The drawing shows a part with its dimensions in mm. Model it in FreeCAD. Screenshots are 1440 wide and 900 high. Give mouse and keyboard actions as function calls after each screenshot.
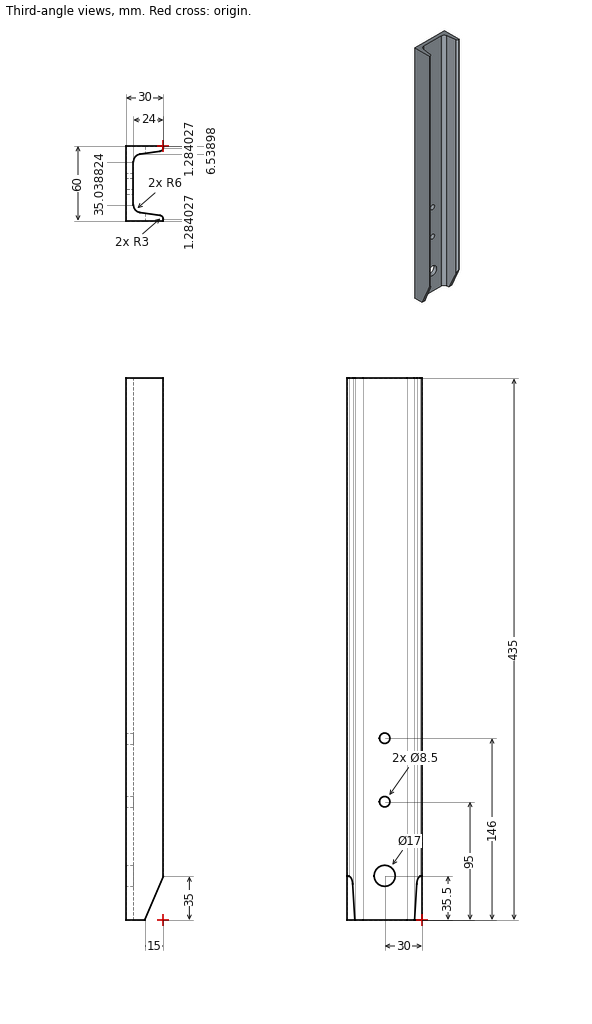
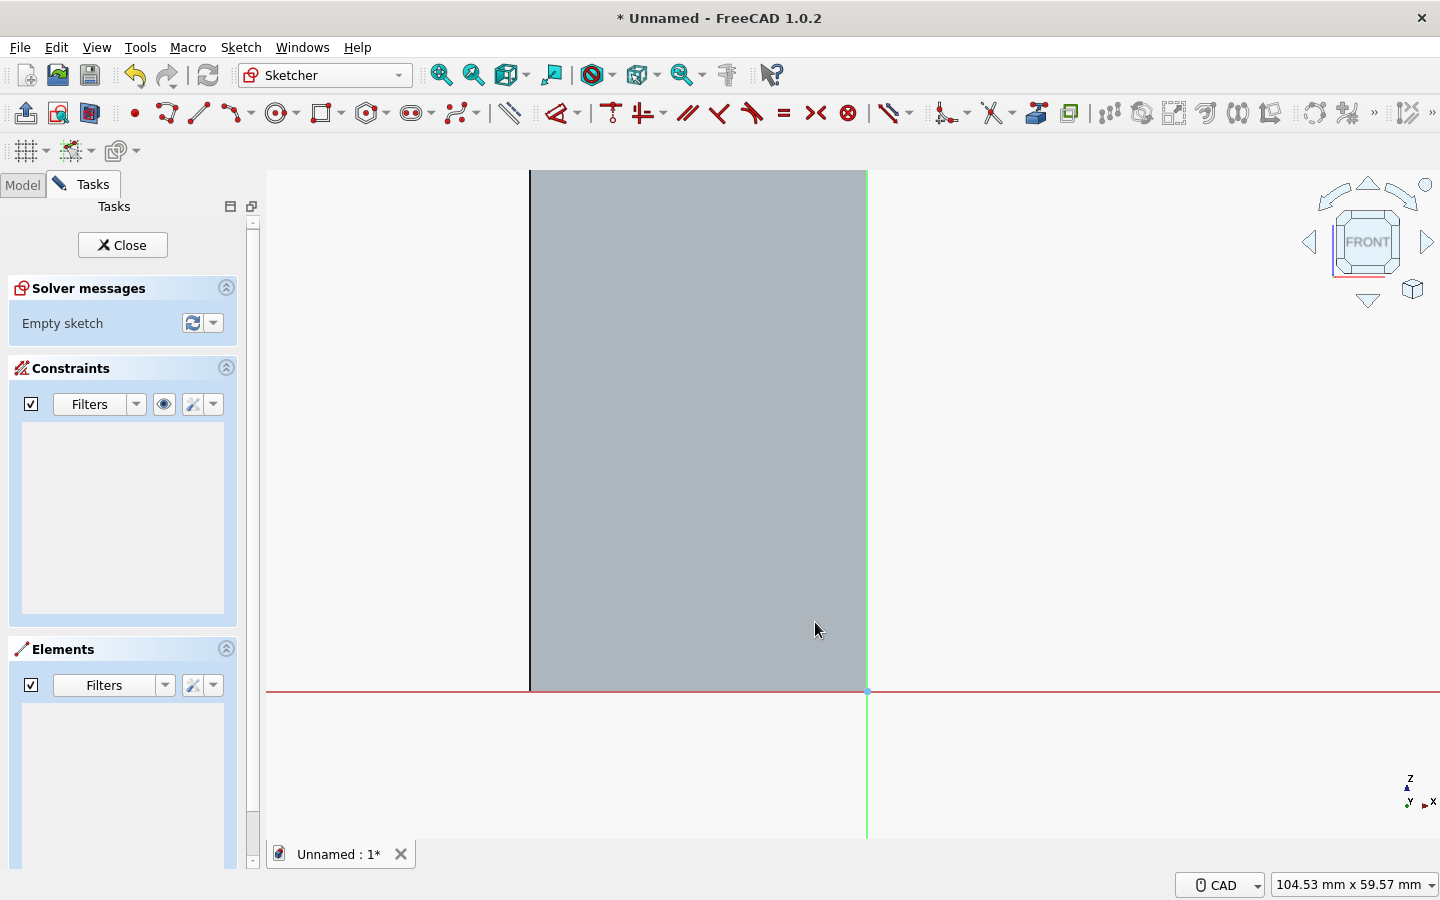
click(168, 114)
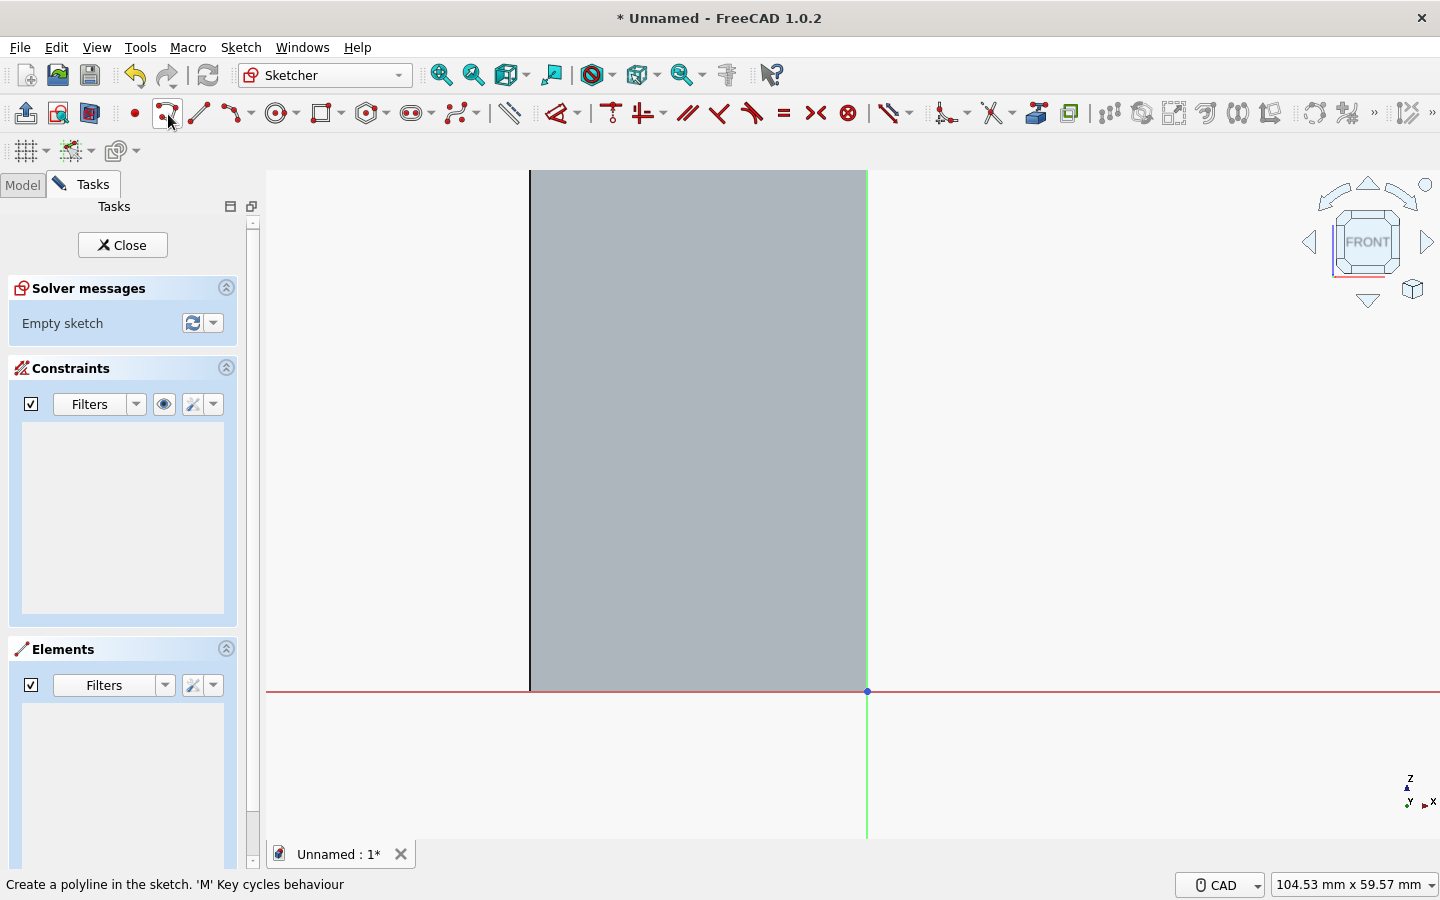
click(867, 692)
click(699, 683)
click(858, 299)
click(867, 692)
key(Escape)
key(Escape)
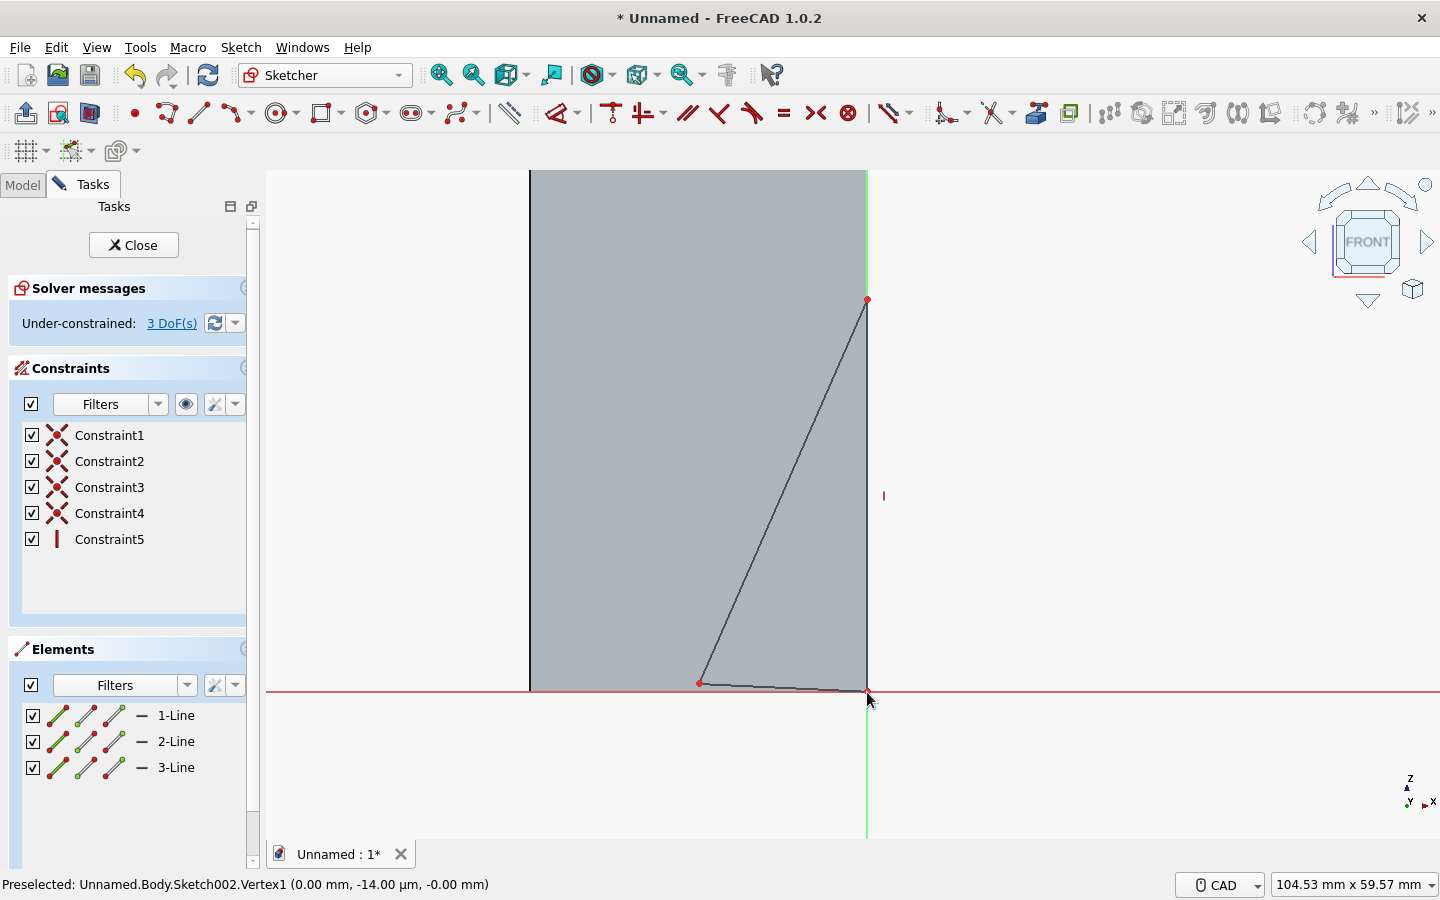
click(817, 689)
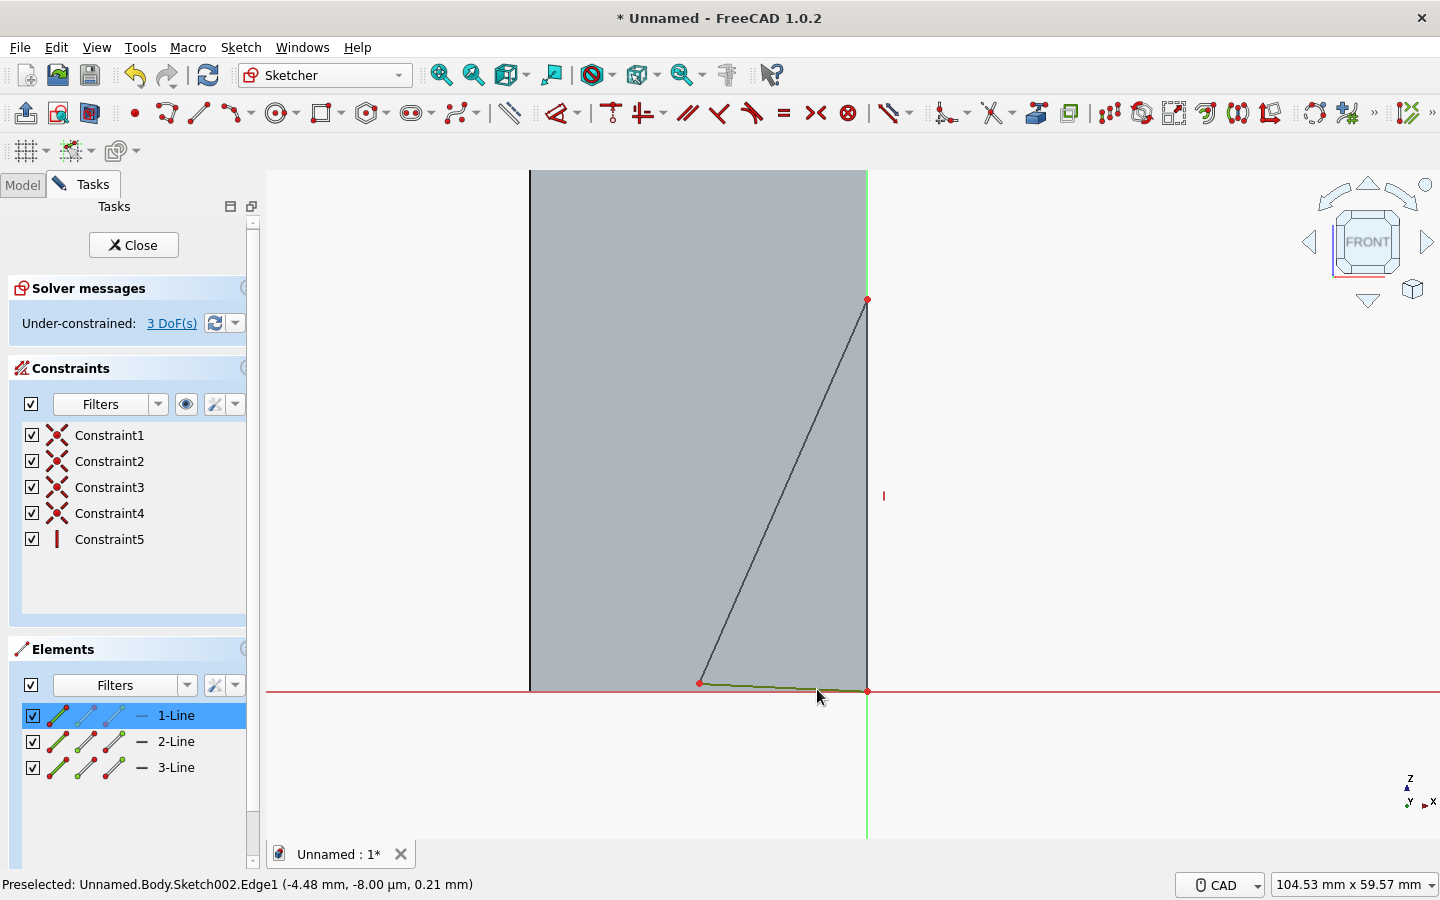
key(h)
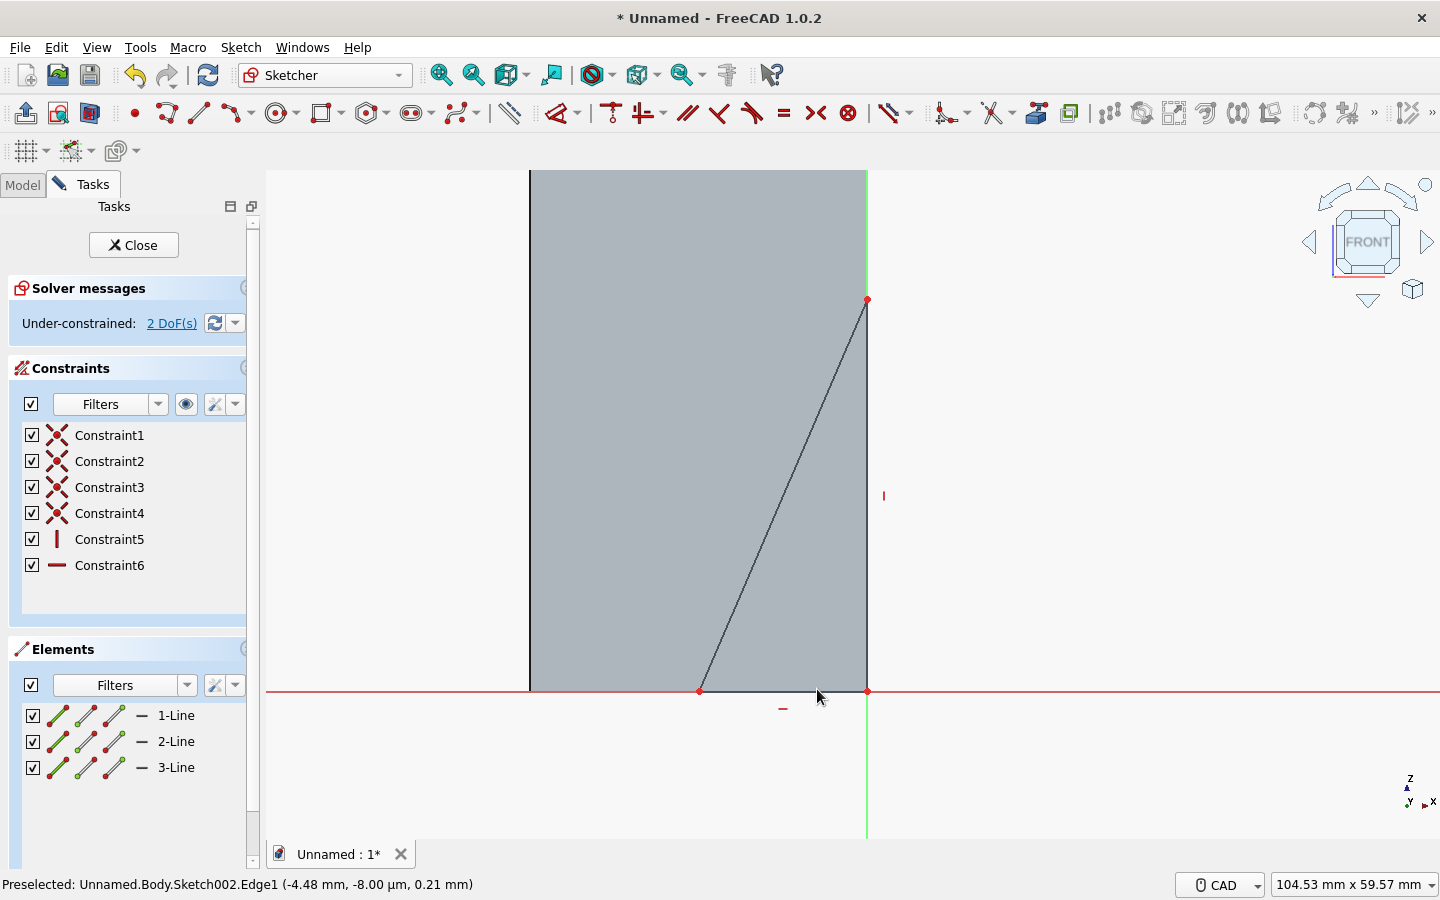
key(d)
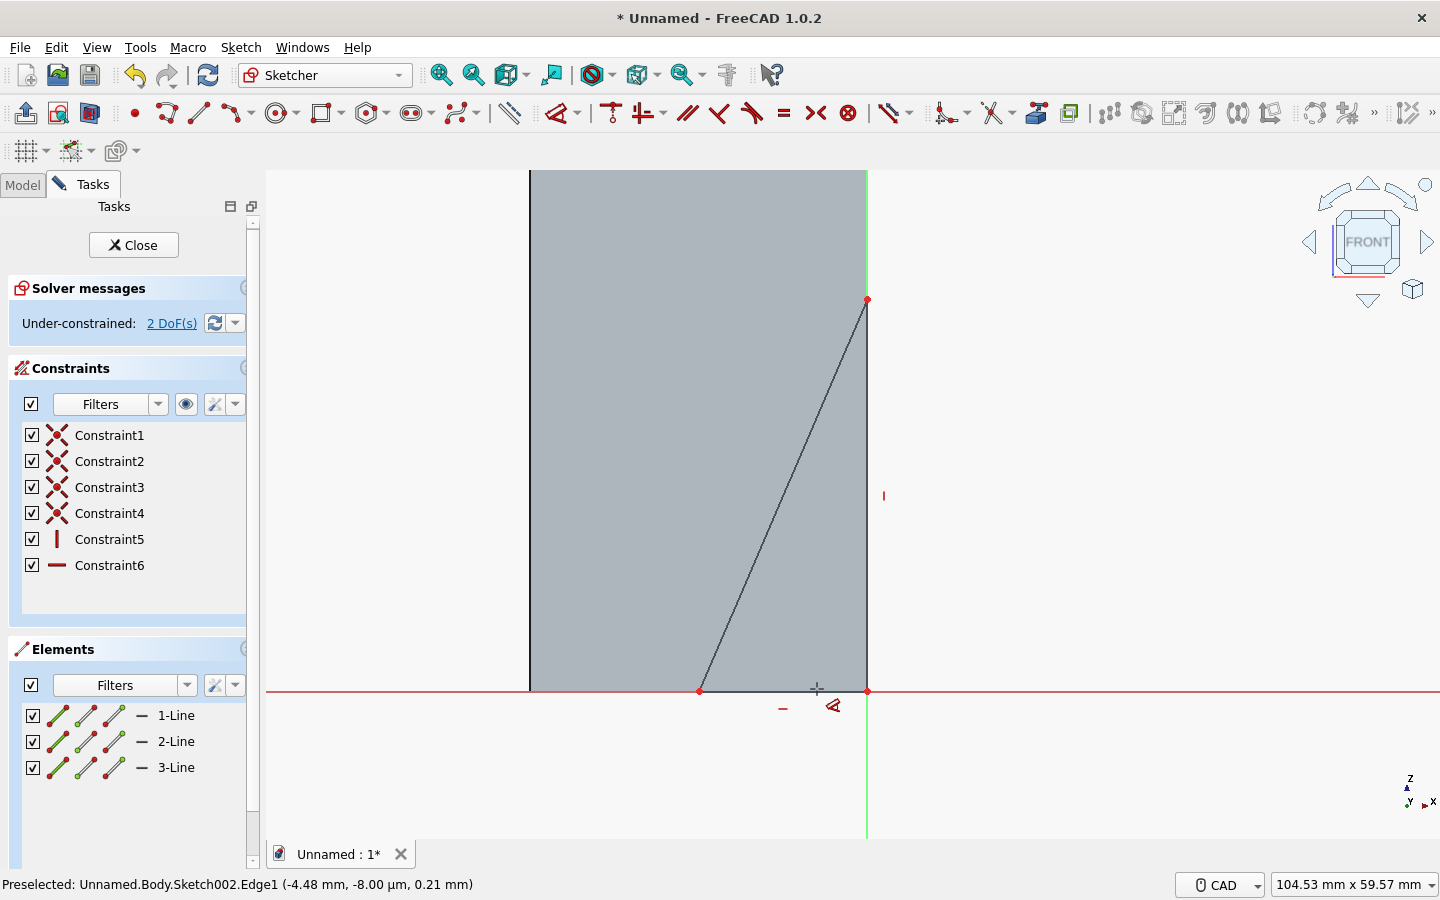
click(817, 692)
click(783, 726)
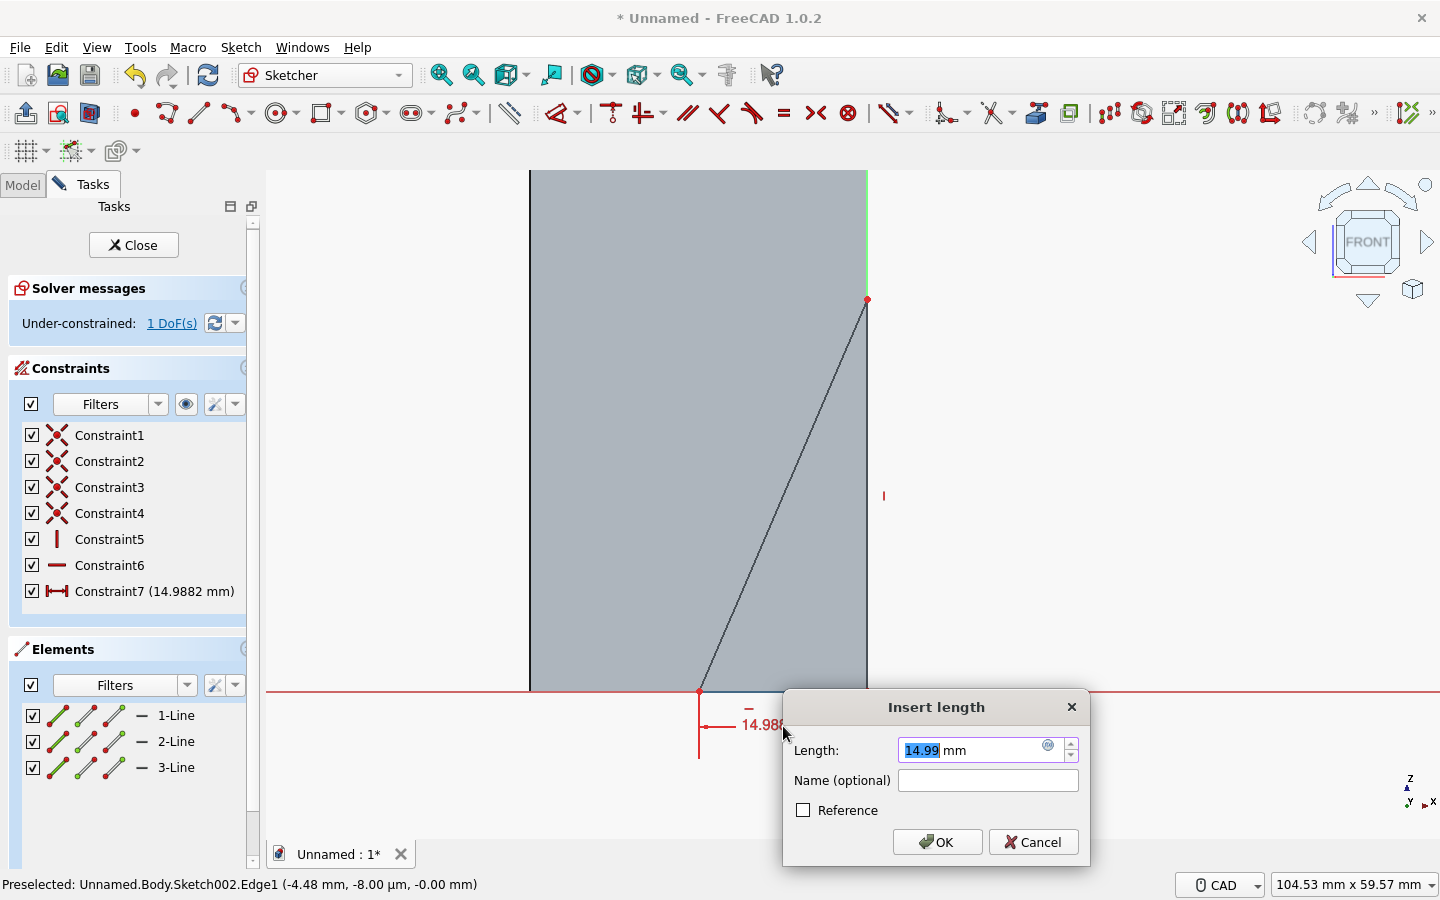
text(15)
key(Return)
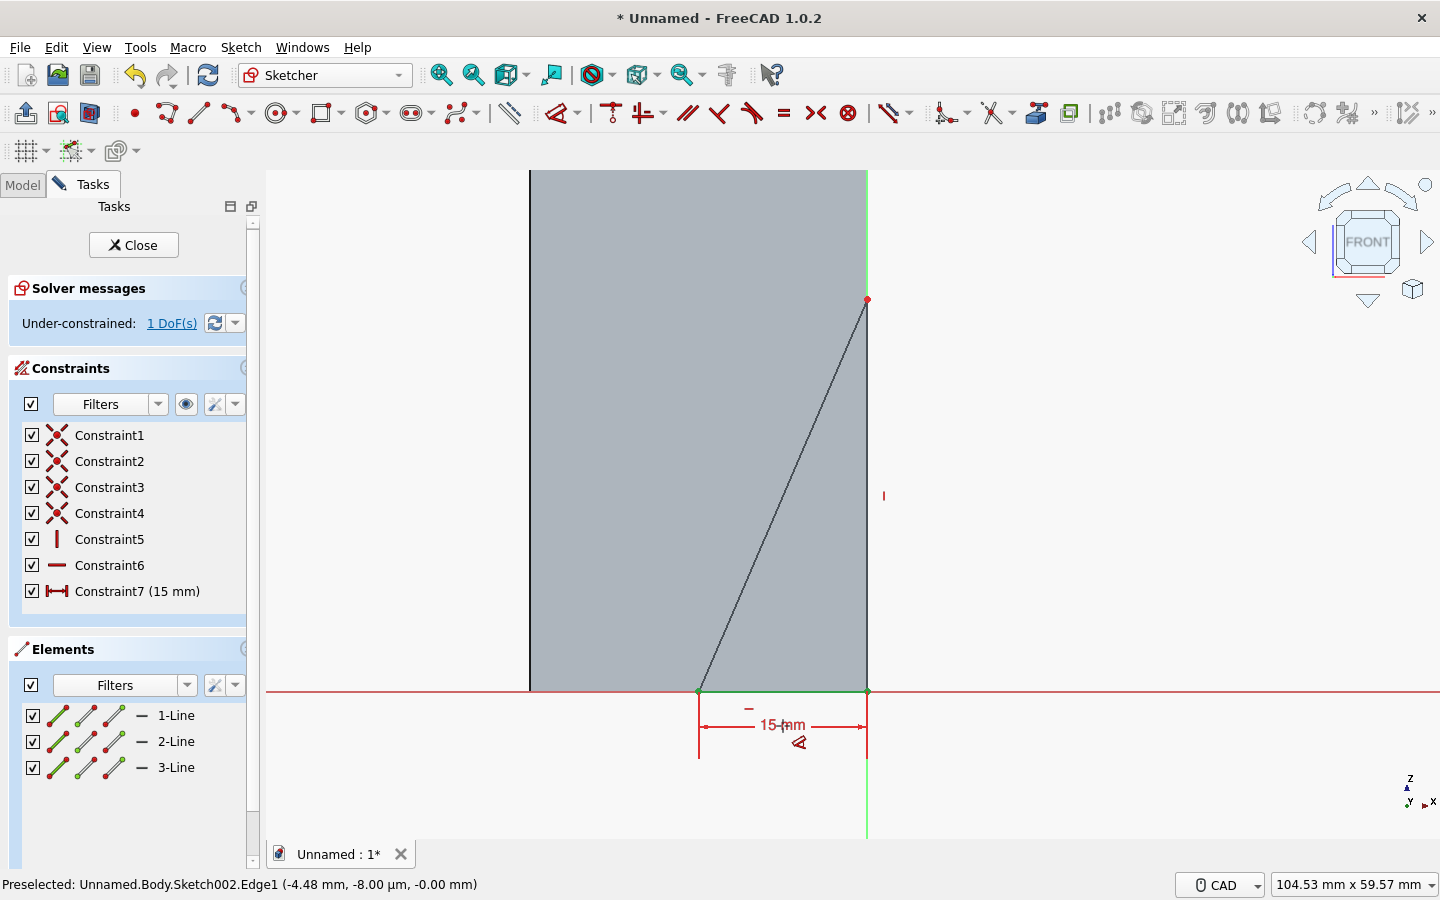
click(867, 418)
click(901, 496)